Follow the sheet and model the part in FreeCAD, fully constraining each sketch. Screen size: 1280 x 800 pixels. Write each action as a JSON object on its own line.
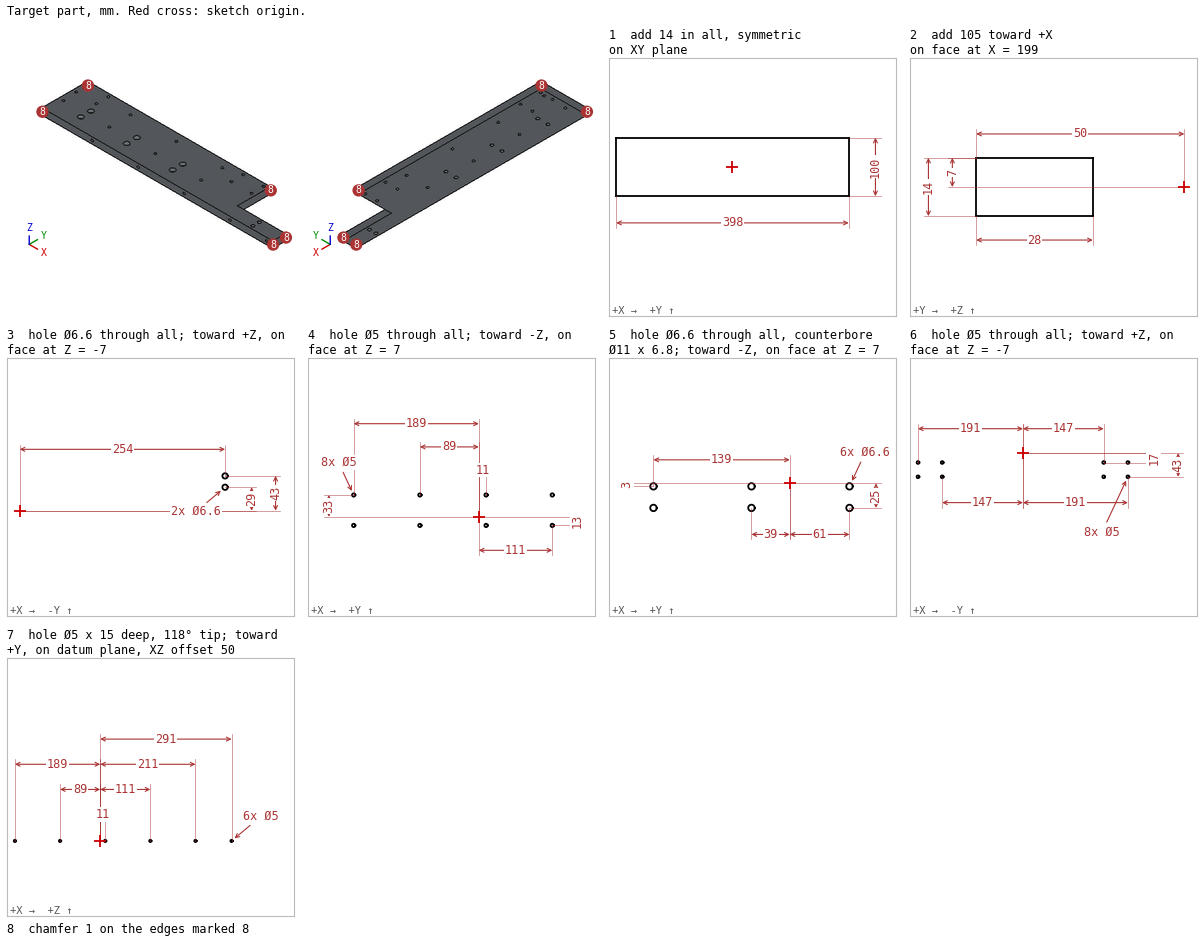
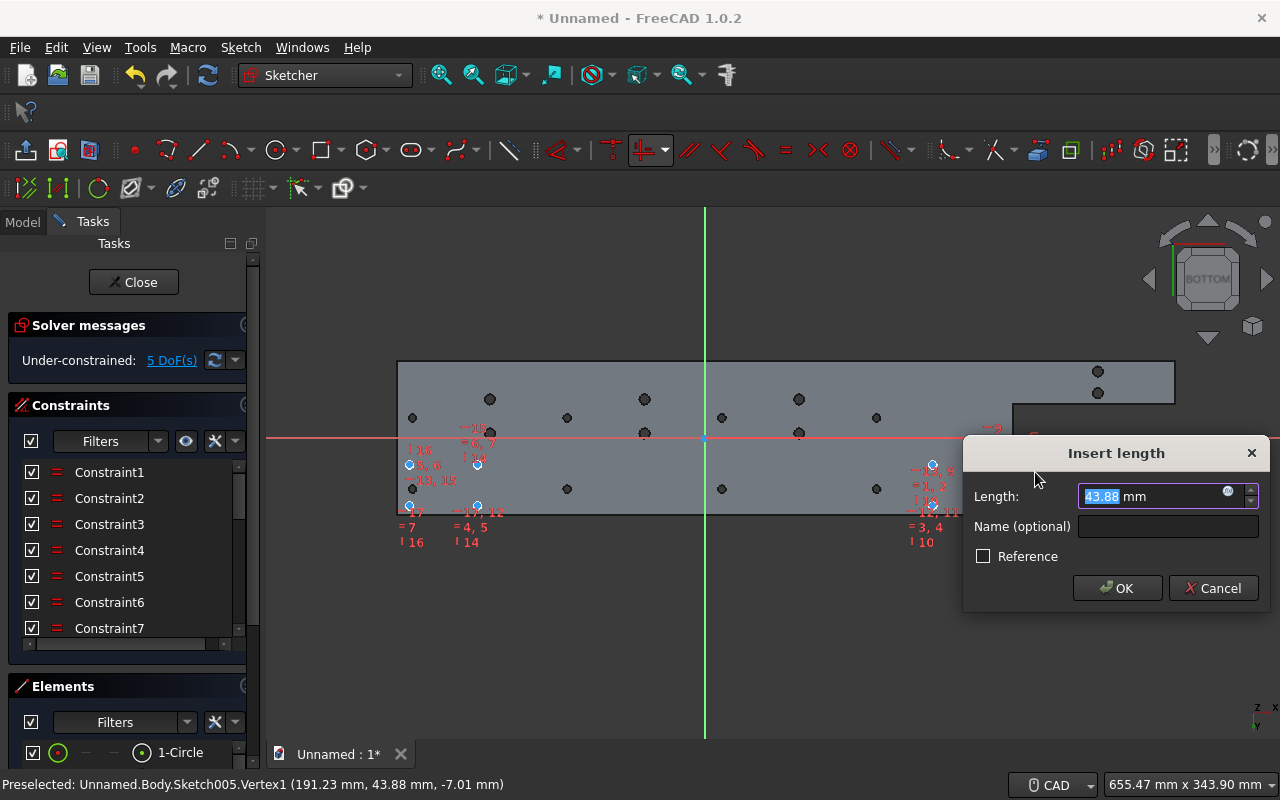
{"action": "type", "text": "43"}
{"action": "key", "text": "Return"}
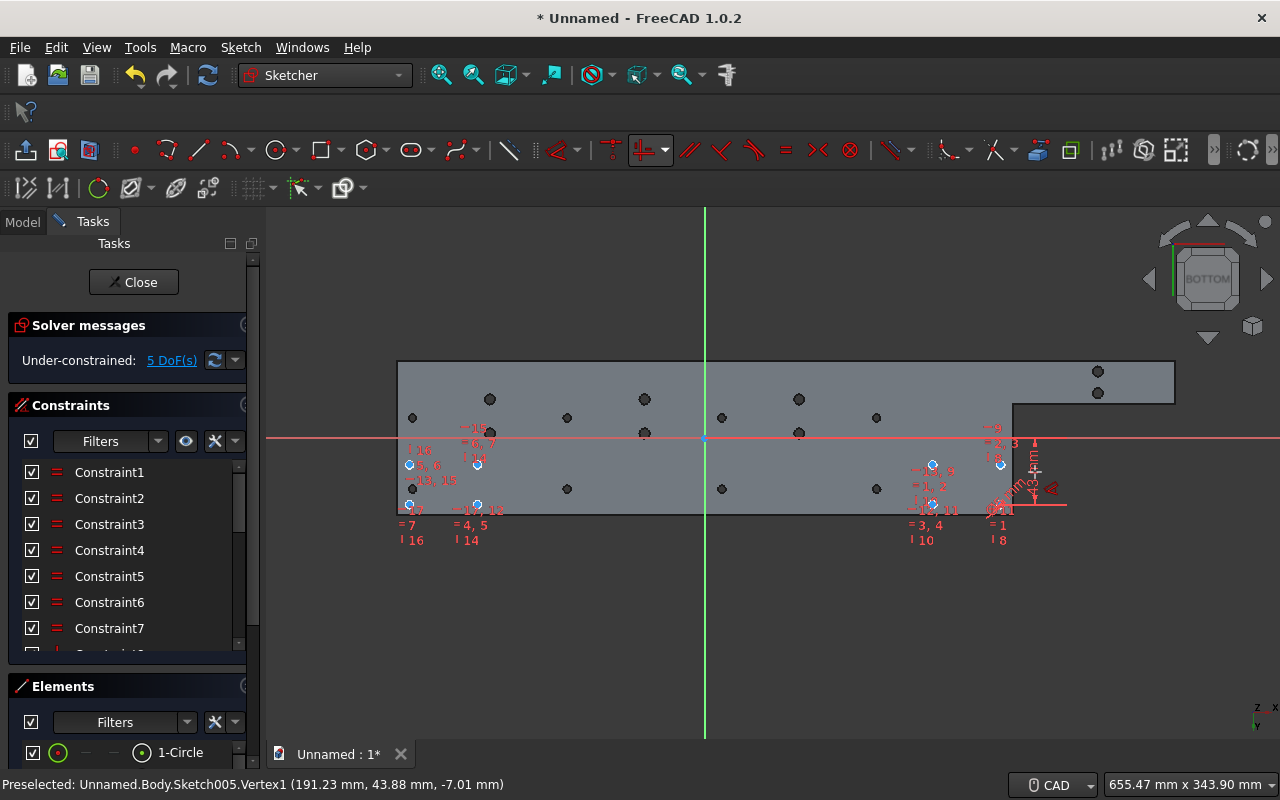
{"action": "scroll", "coordinate": [933, 465], "scroll_direction": "up", "scroll_amount": 3}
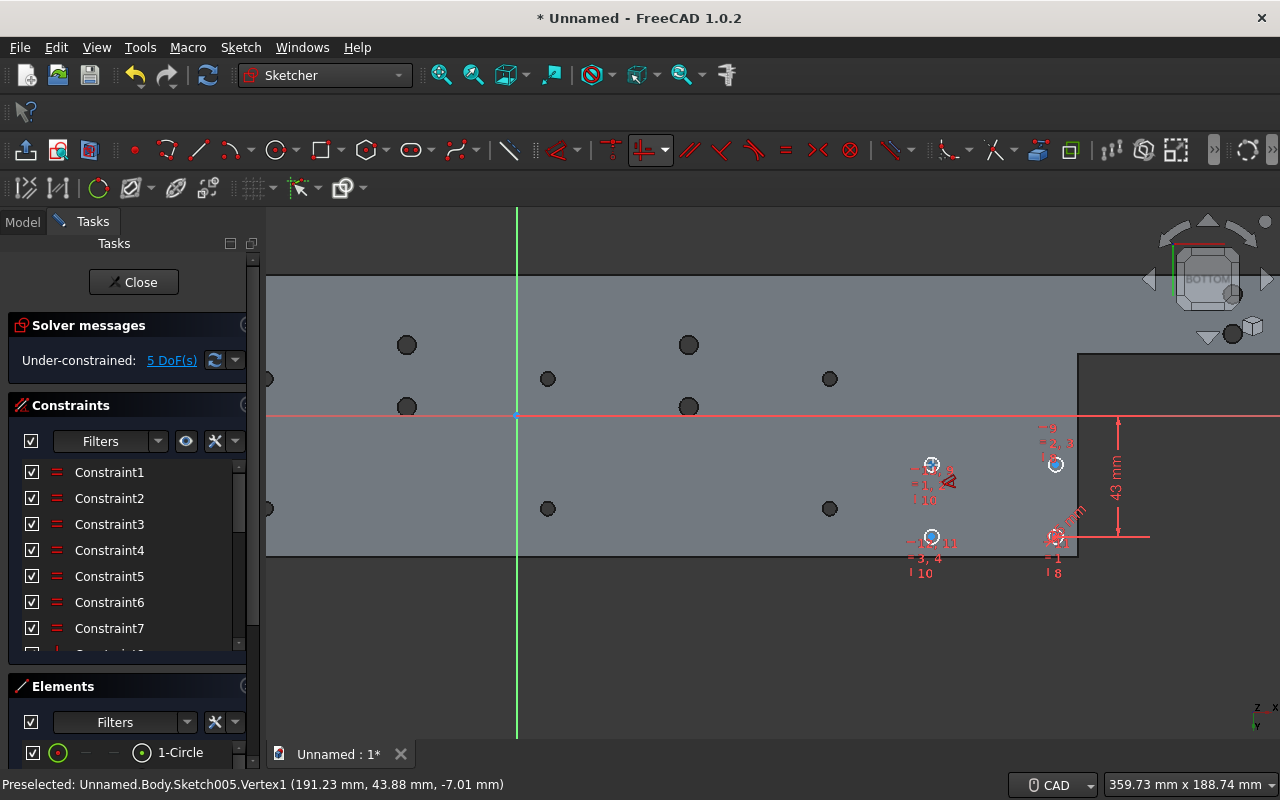
{"action": "left_click", "coordinate": [932, 465]}
{"action": "left_click", "coordinate": [966, 440]}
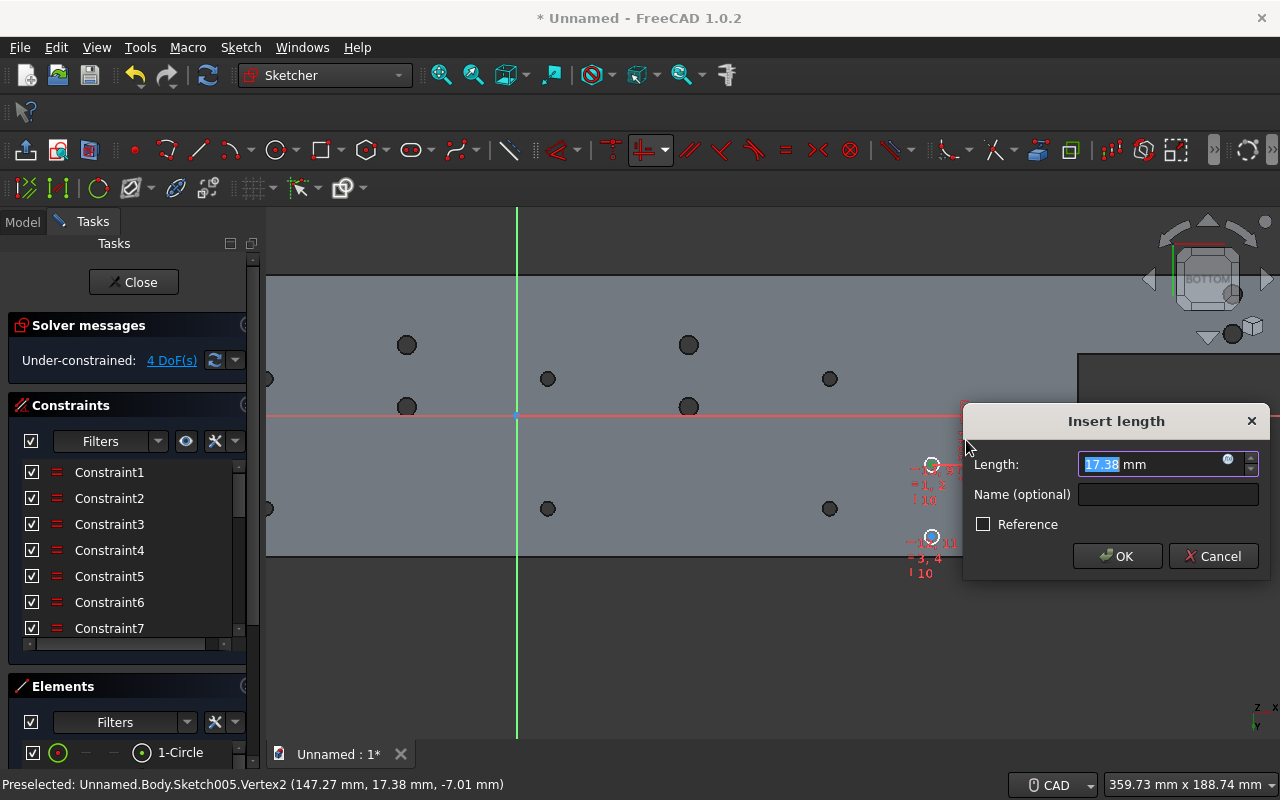
{"action": "type", "text": "17"}
{"action": "key", "text": "Return"}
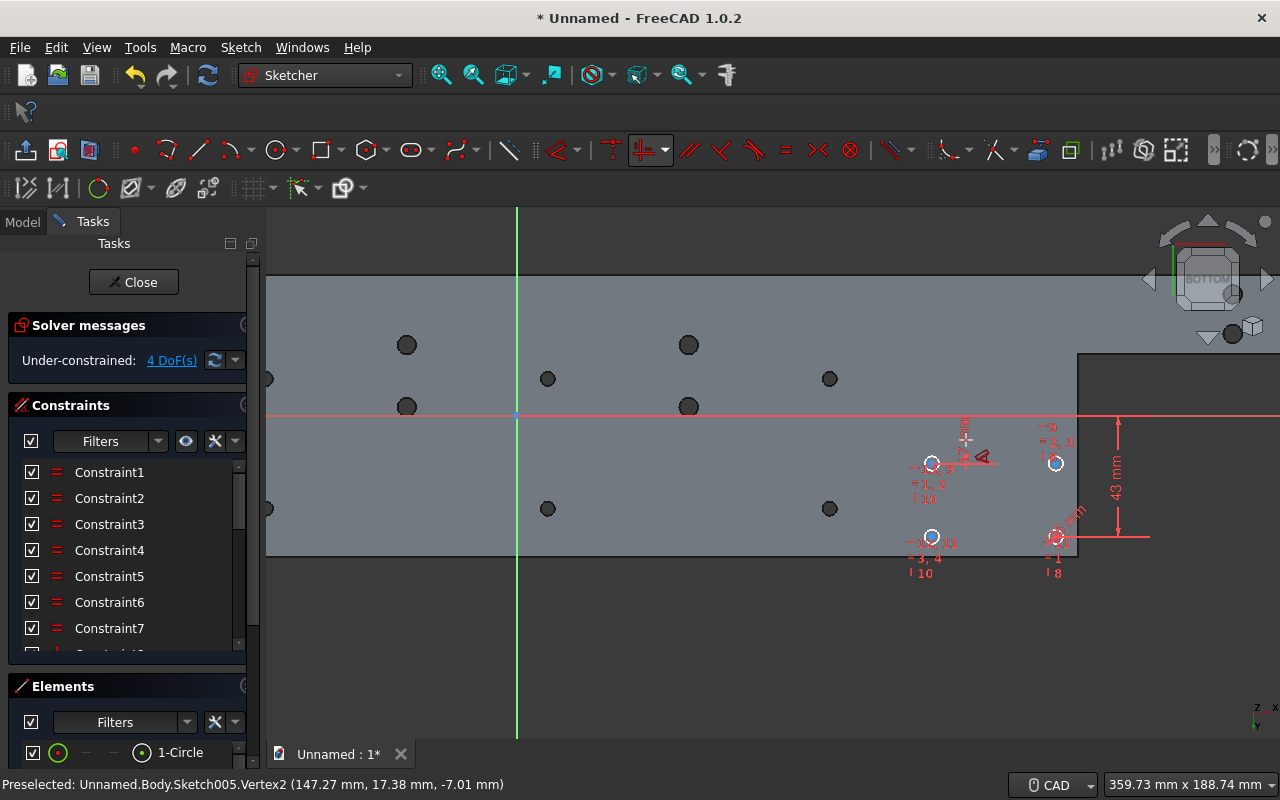
{"action": "left_click", "coordinate": [1056, 537]}
{"action": "left_click", "coordinate": [786, 382]}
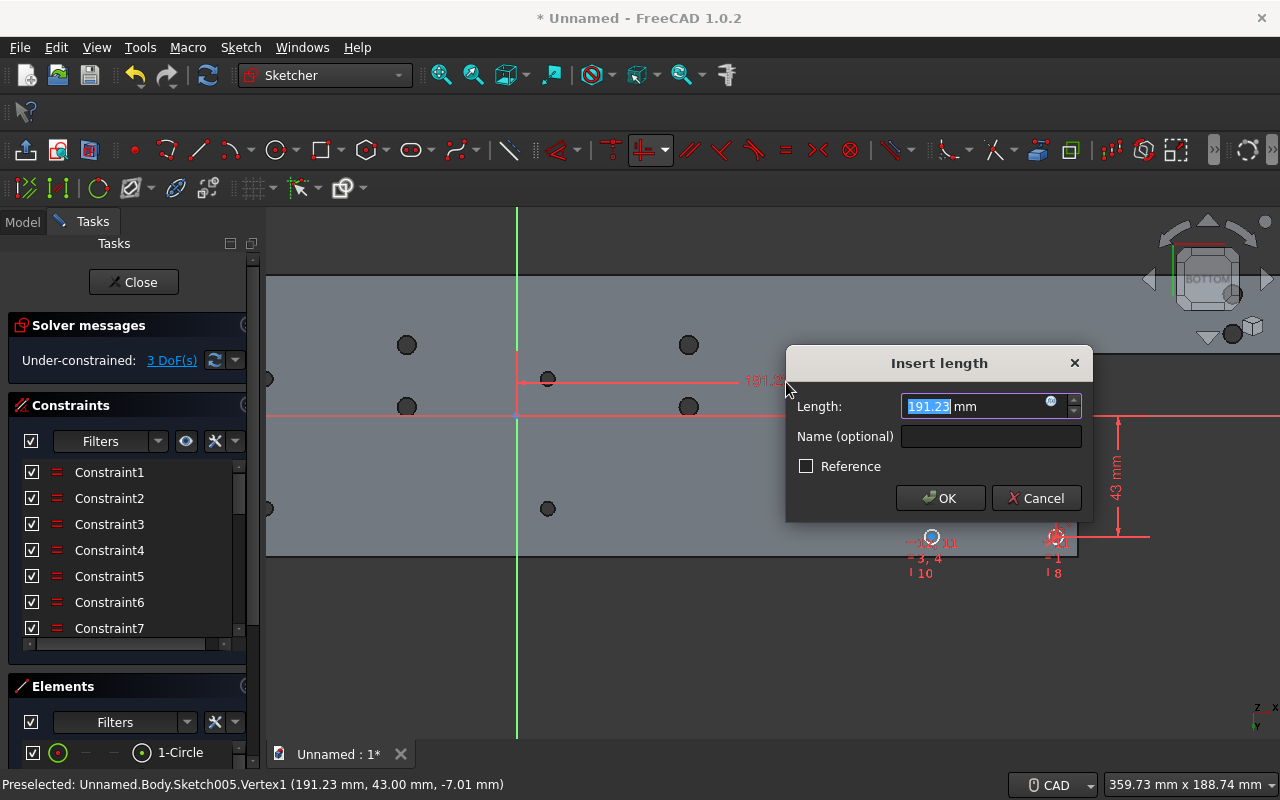
{"action": "type", "text": "191"}
{"action": "key", "text": "Return"}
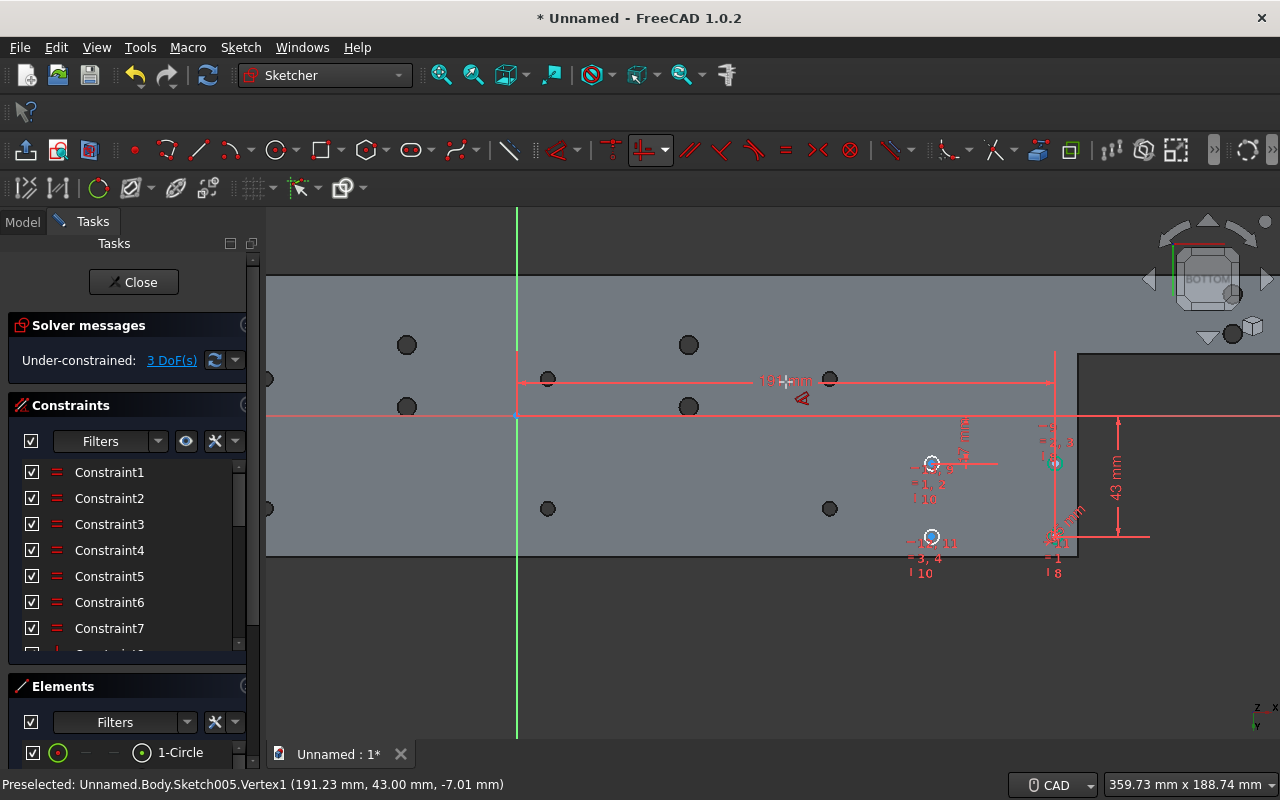
{"action": "left_click", "coordinate": [932, 464]}
{"action": "left_click", "coordinate": [629, 382]}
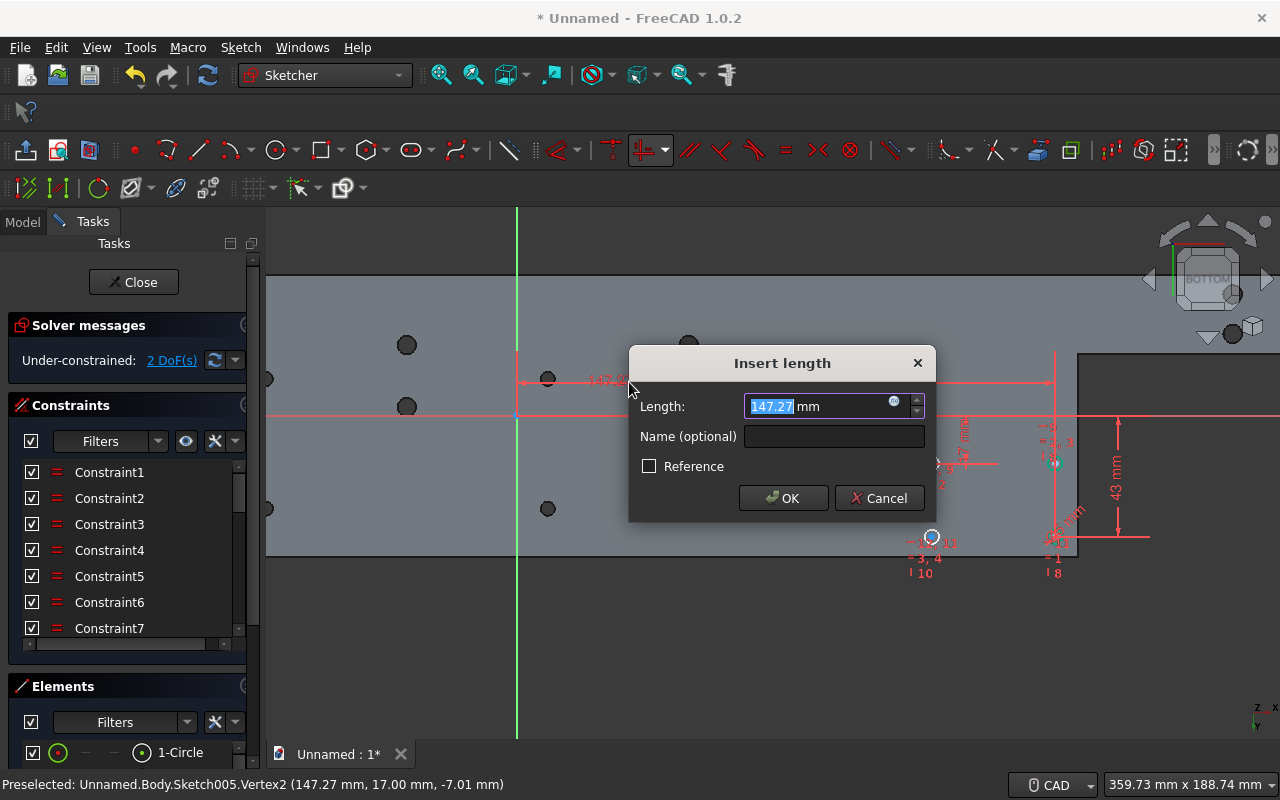
{"action": "type", "text": "147"}
{"action": "key", "text": "Return"}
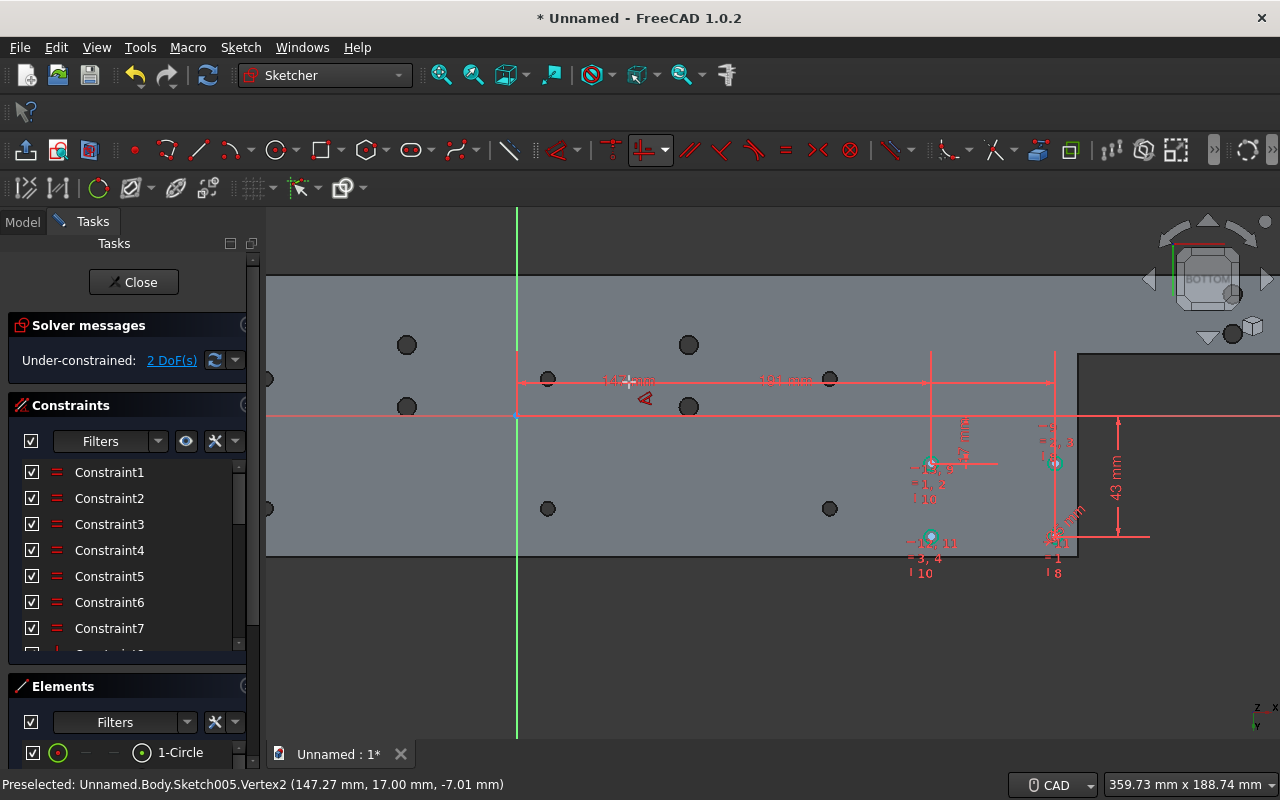
{"action": "scroll", "coordinate": [933, 465], "scroll_direction": "down", "scroll_amount": 3}